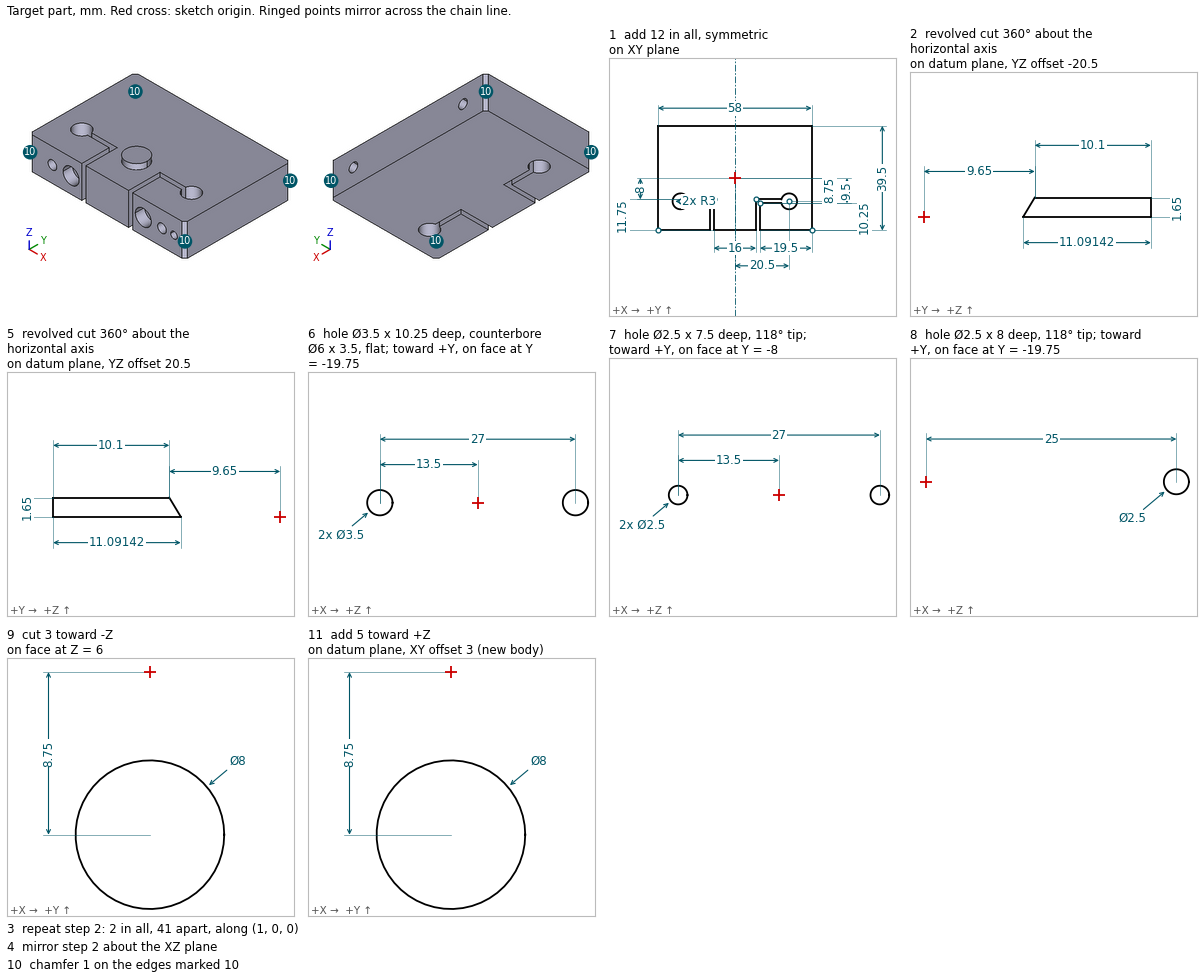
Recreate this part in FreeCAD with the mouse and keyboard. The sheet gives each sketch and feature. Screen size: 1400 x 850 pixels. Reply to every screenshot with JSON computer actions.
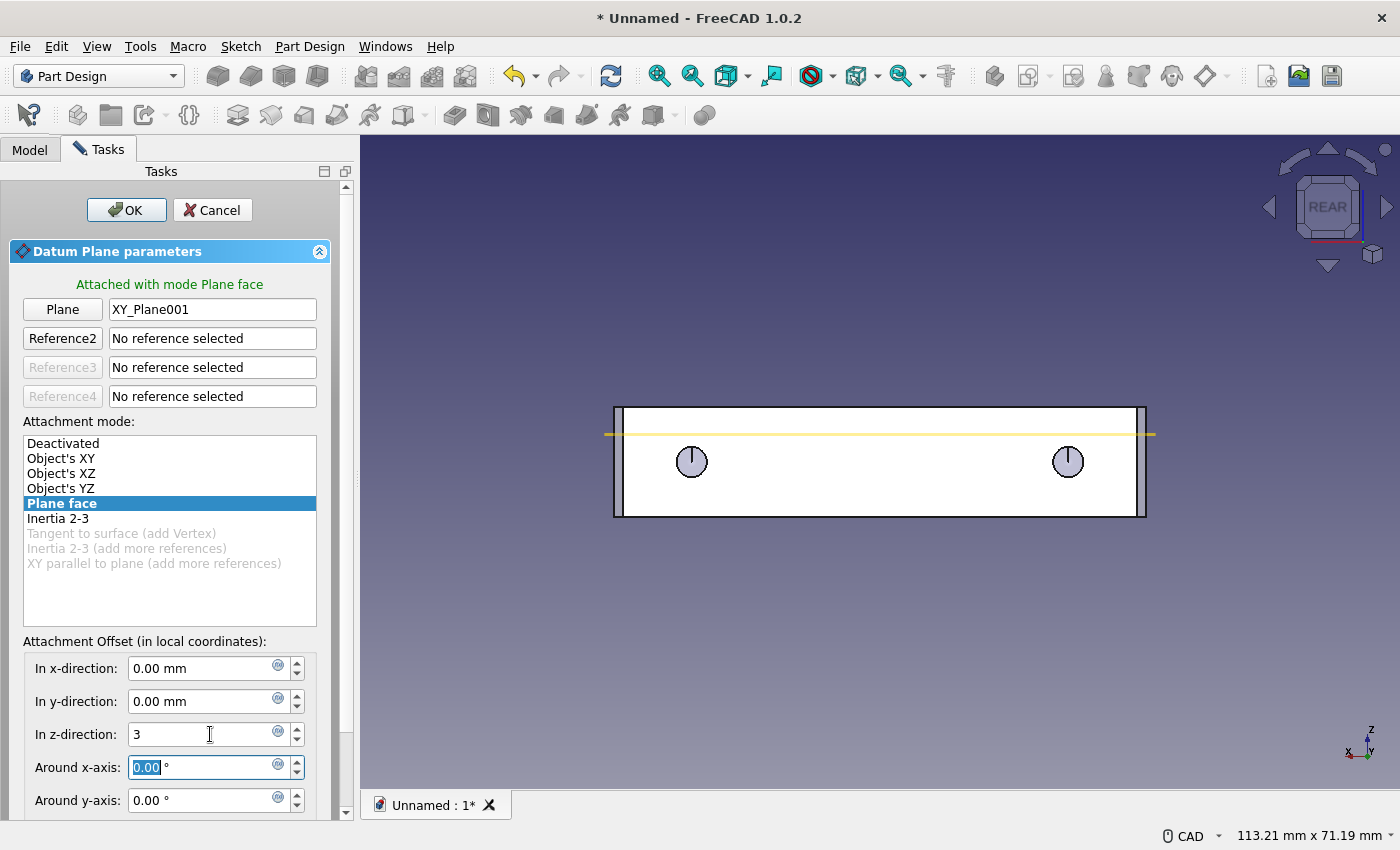
{"action": "left_click", "coordinate": [127, 210]}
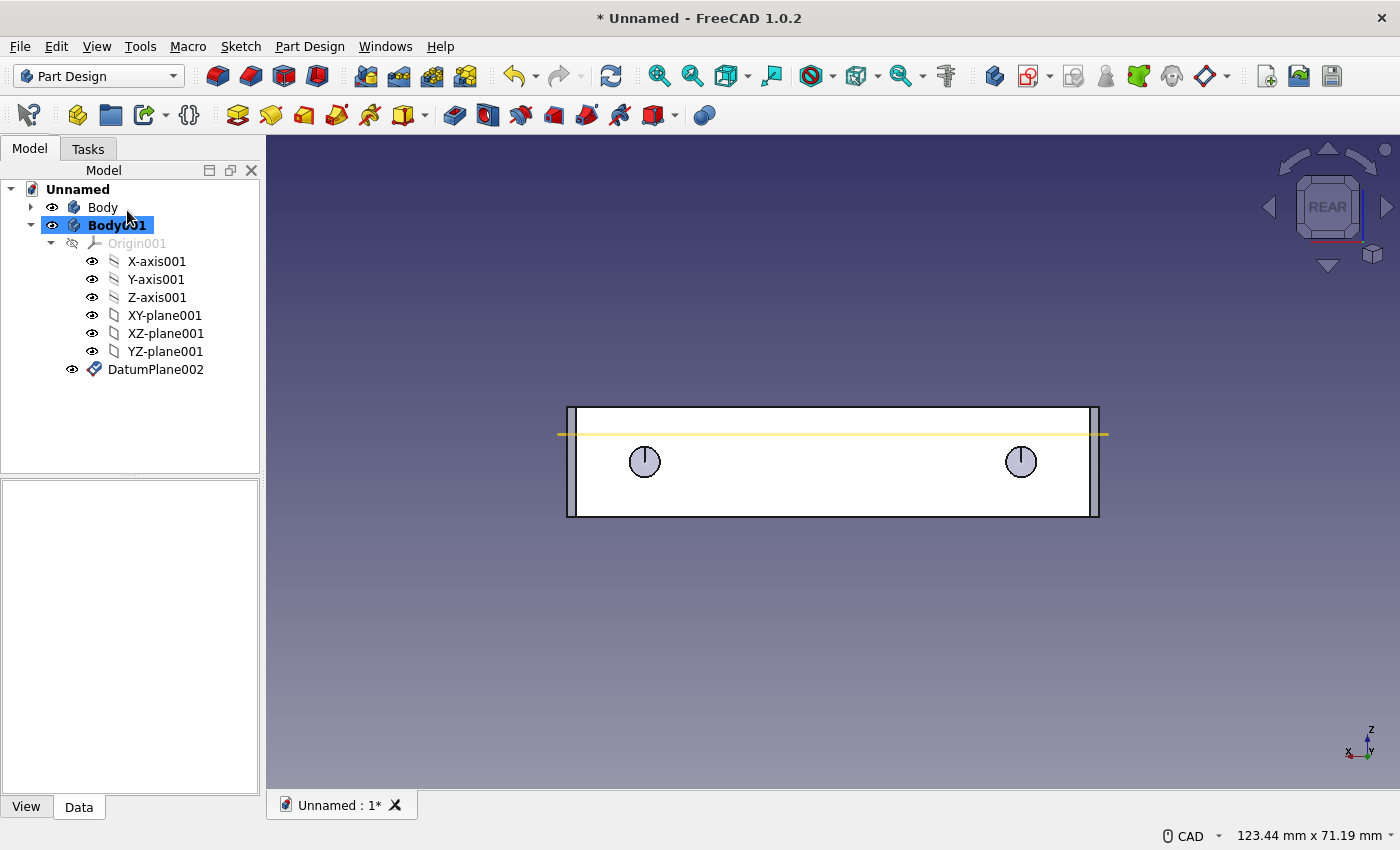
{"action": "left_click", "coordinate": [117, 369]}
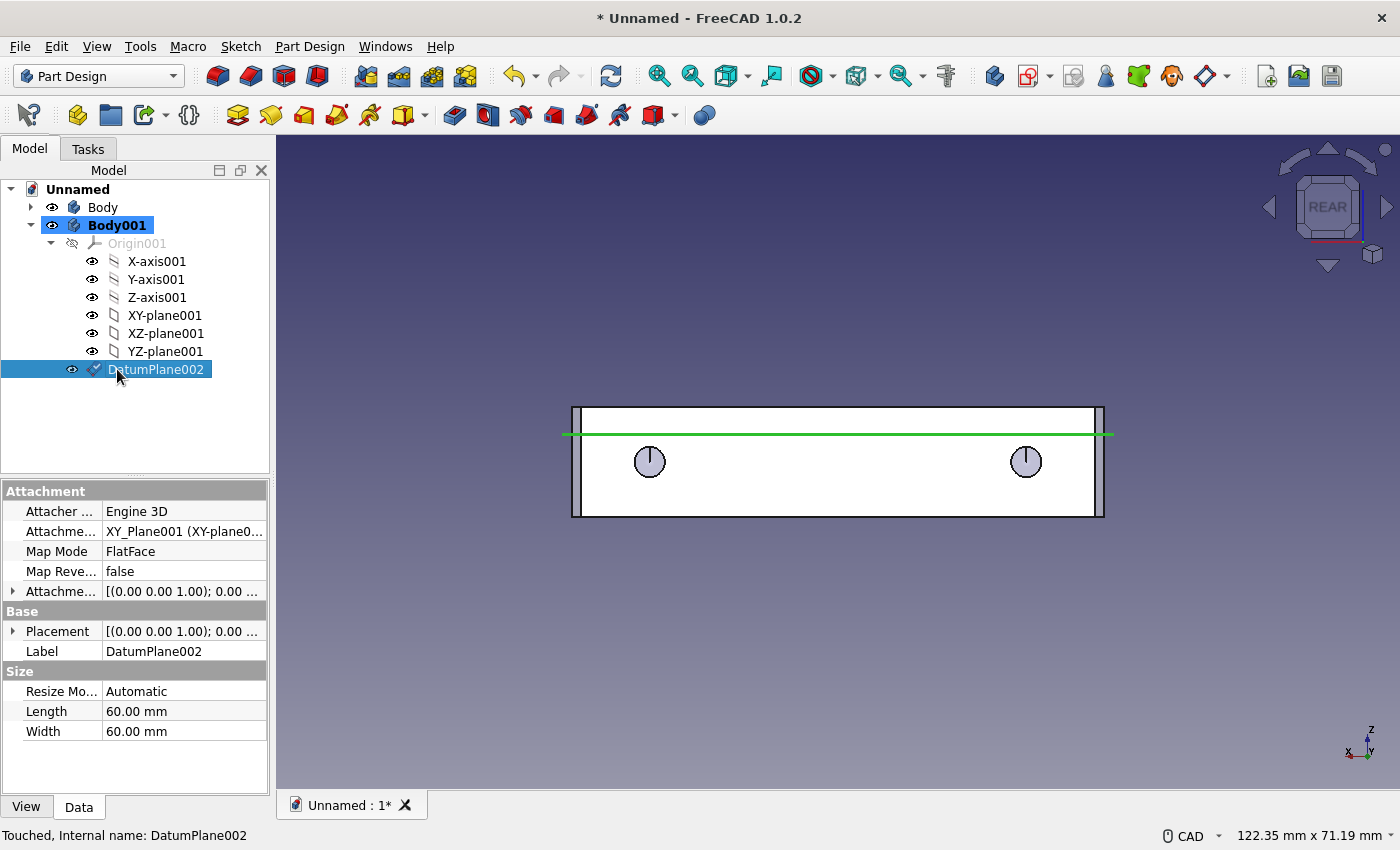
{"action": "left_click", "coordinate": [1028, 76]}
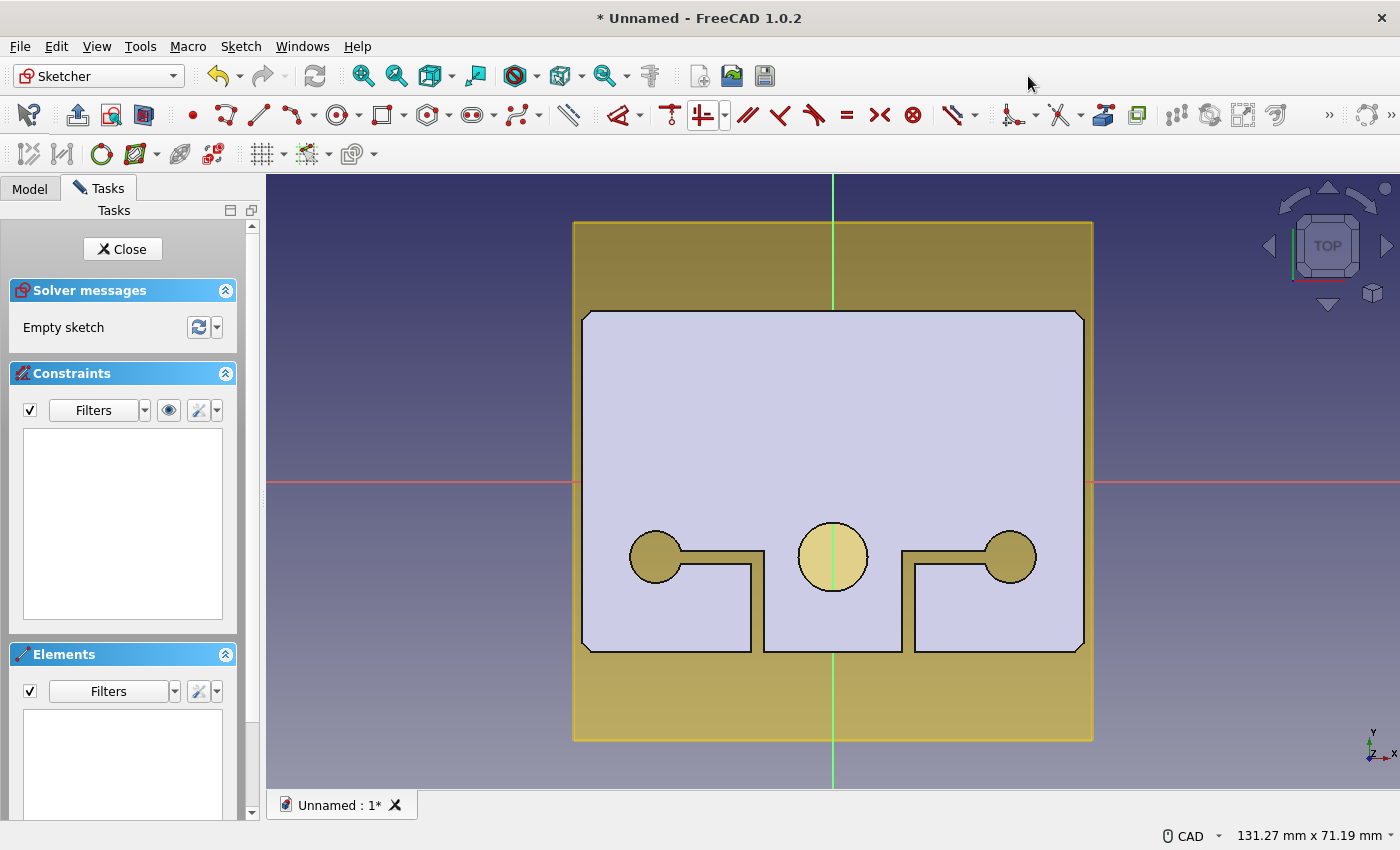
{"action": "scroll", "coordinate": [863, 560], "scroll_direction": "up", "scroll_amount": 6}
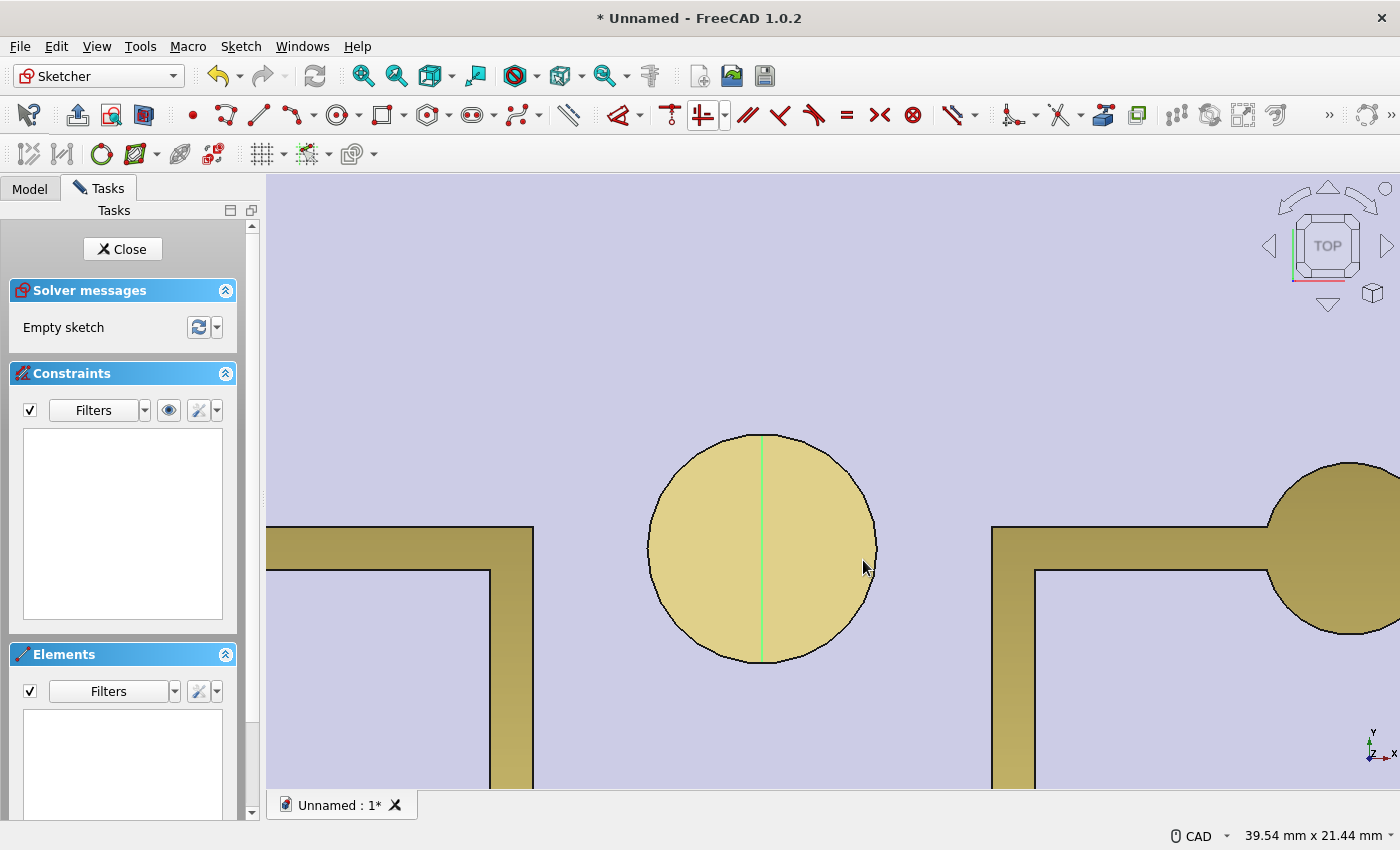
{"action": "left_click", "coordinate": [336, 116]}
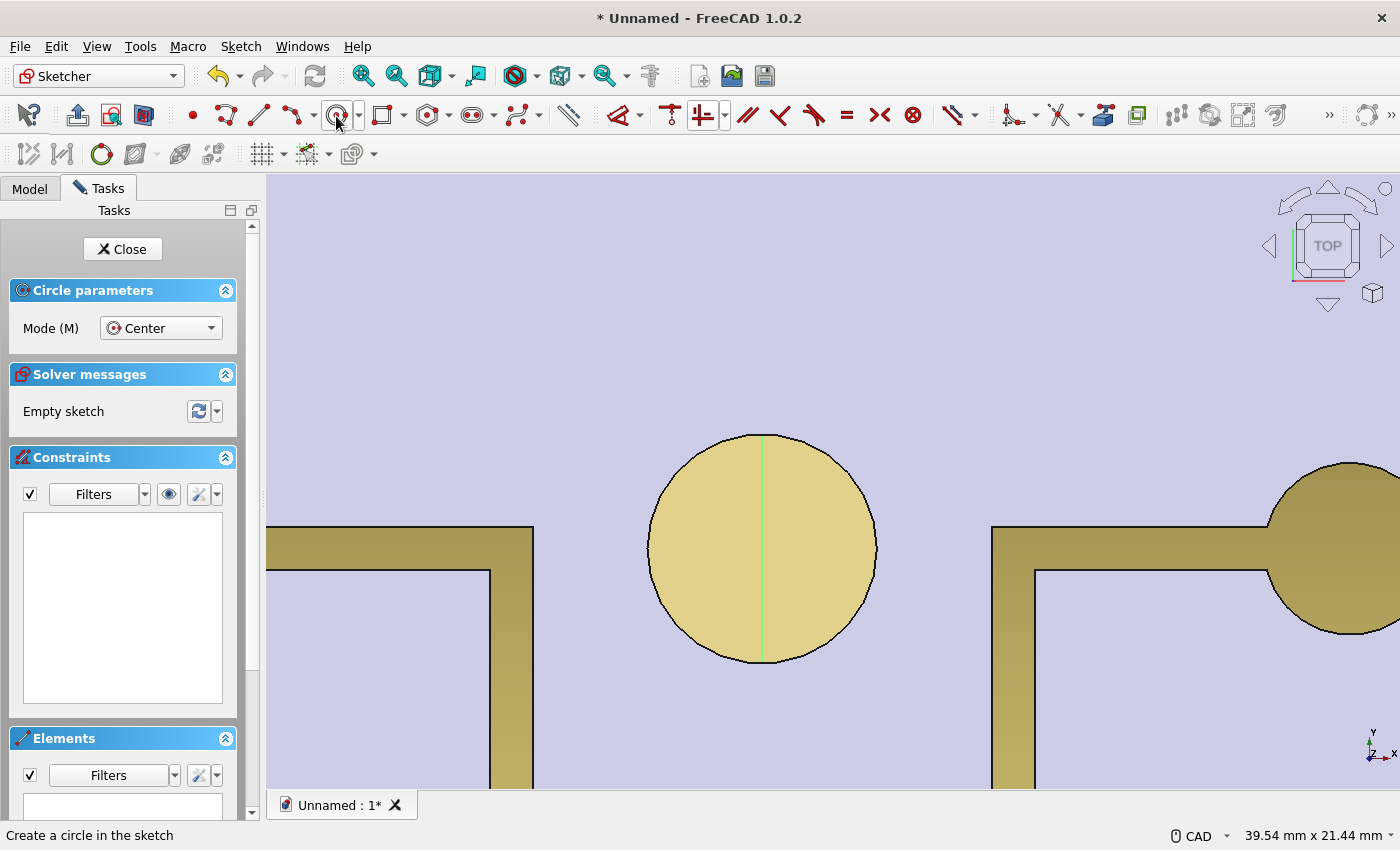
{"action": "left_click", "coordinate": [762, 549]}
{"action": "left_click", "coordinate": [843, 468]}
{"action": "key", "text": "Escape"}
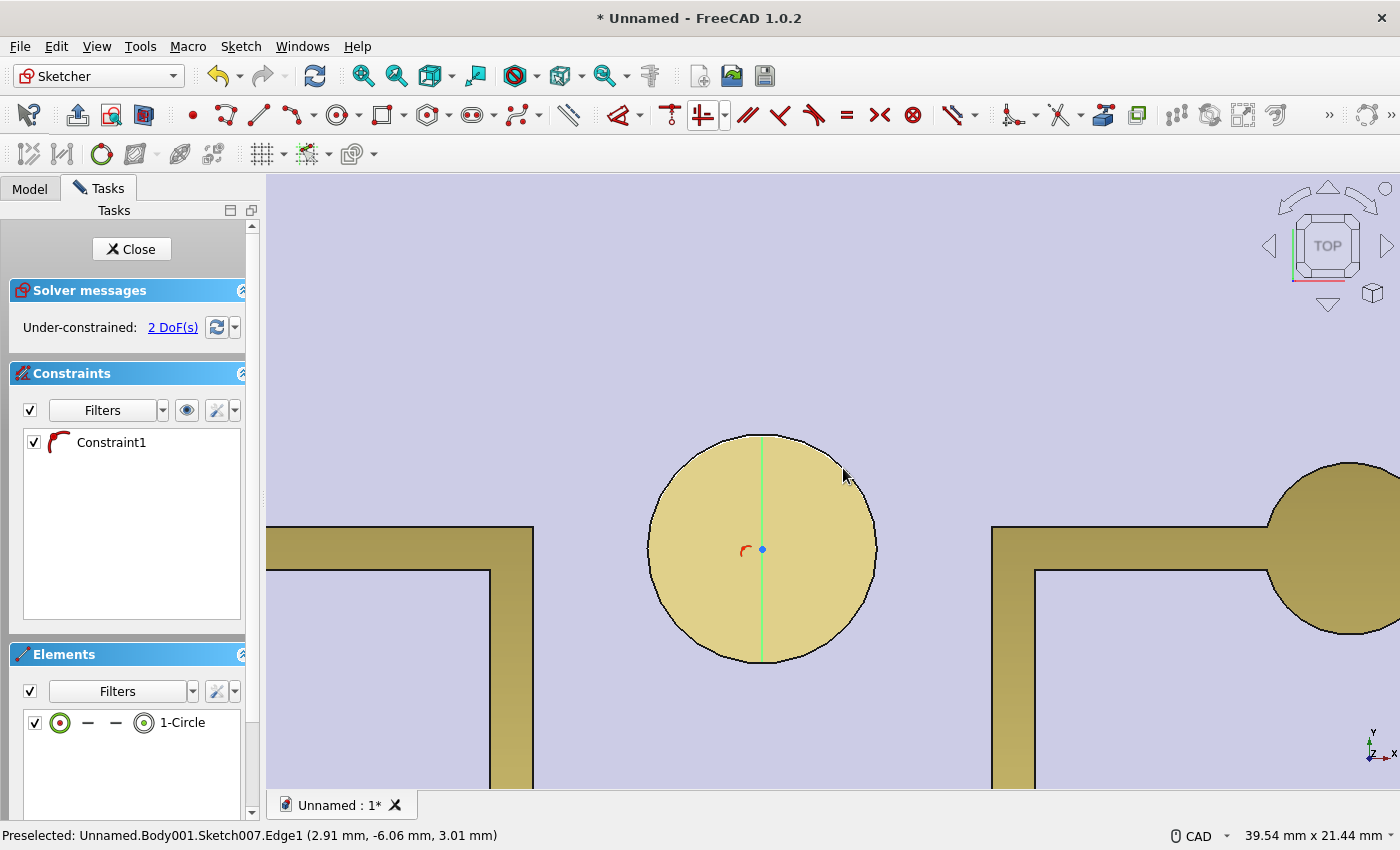
{"action": "key", "text": "d"}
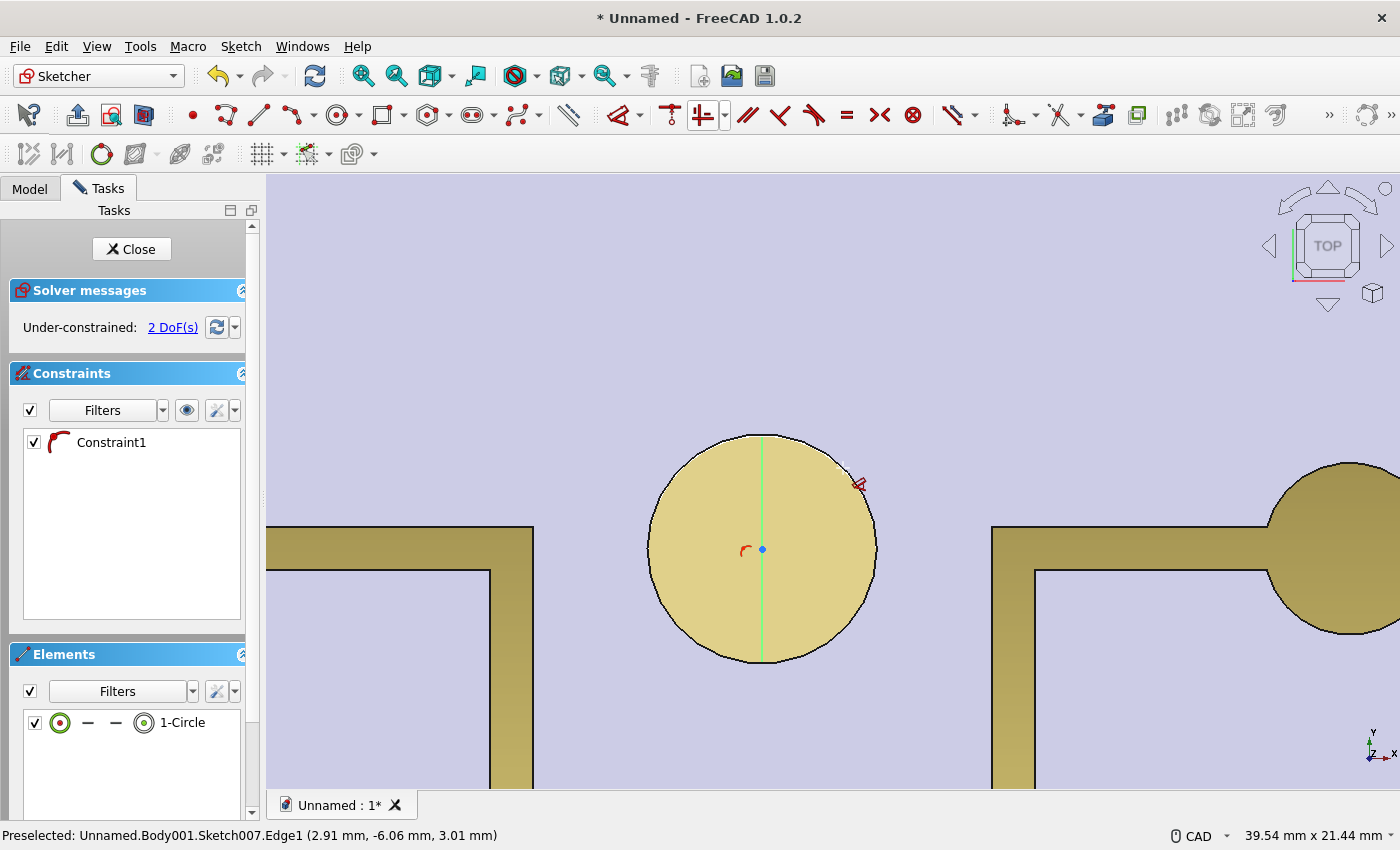
{"action": "left_click", "coordinate": [843, 469]}
{"action": "left_click", "coordinate": [866, 446]}